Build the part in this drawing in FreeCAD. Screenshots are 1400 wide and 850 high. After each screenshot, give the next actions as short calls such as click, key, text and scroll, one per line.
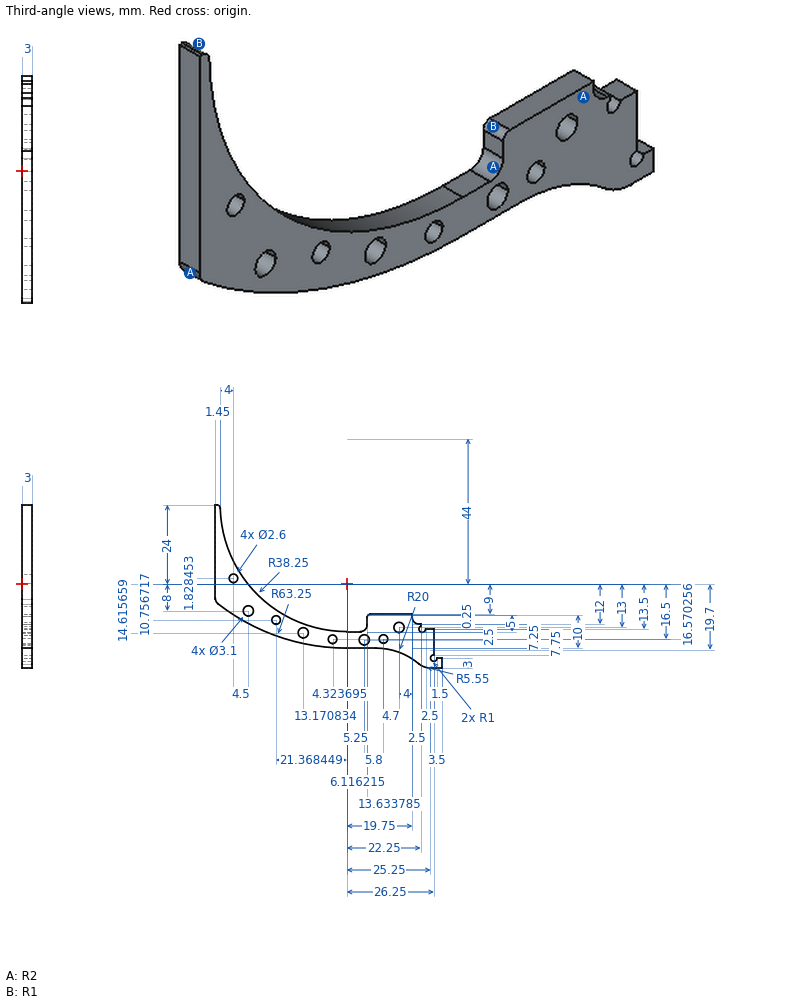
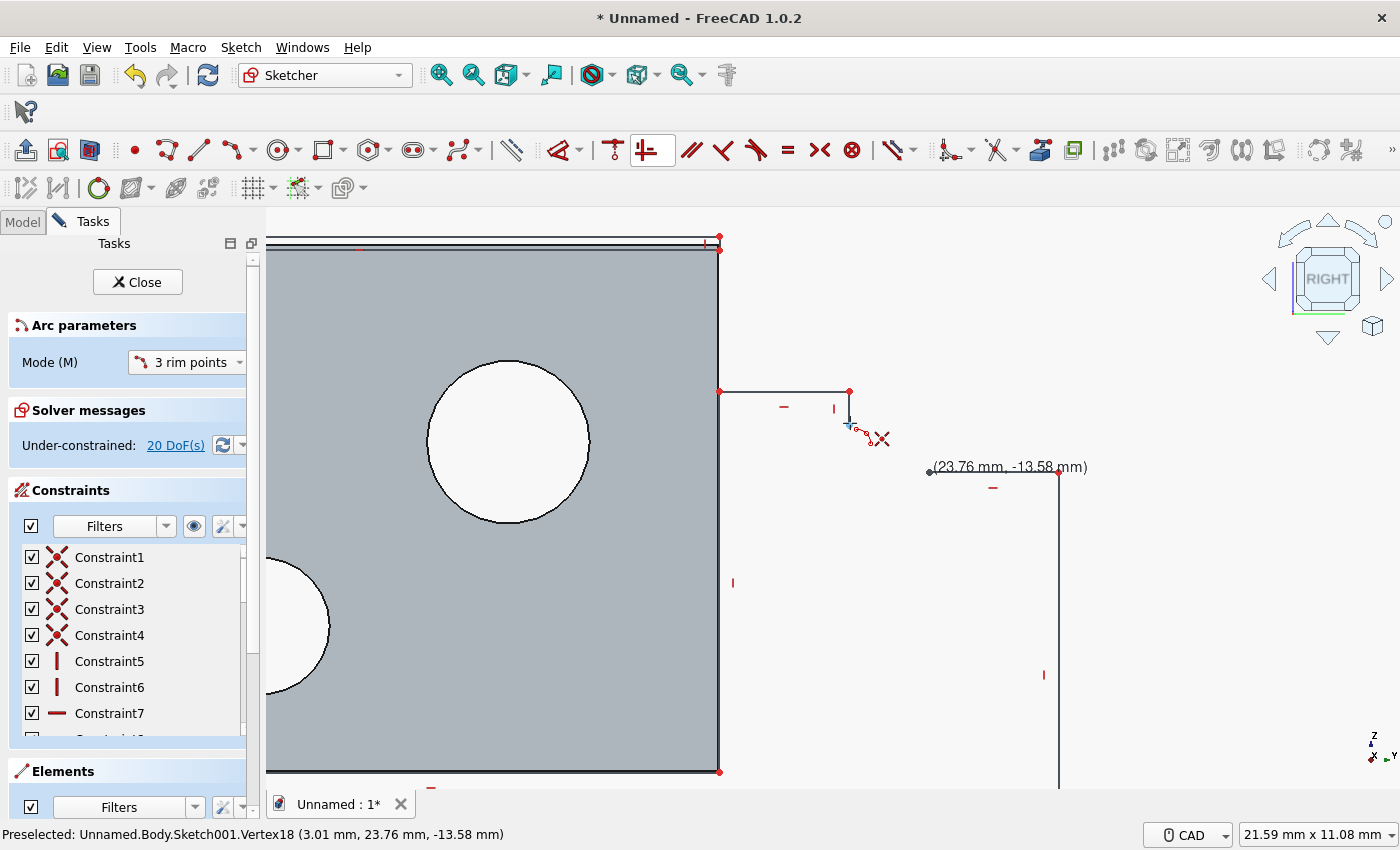
click(849, 426)
click(850, 514)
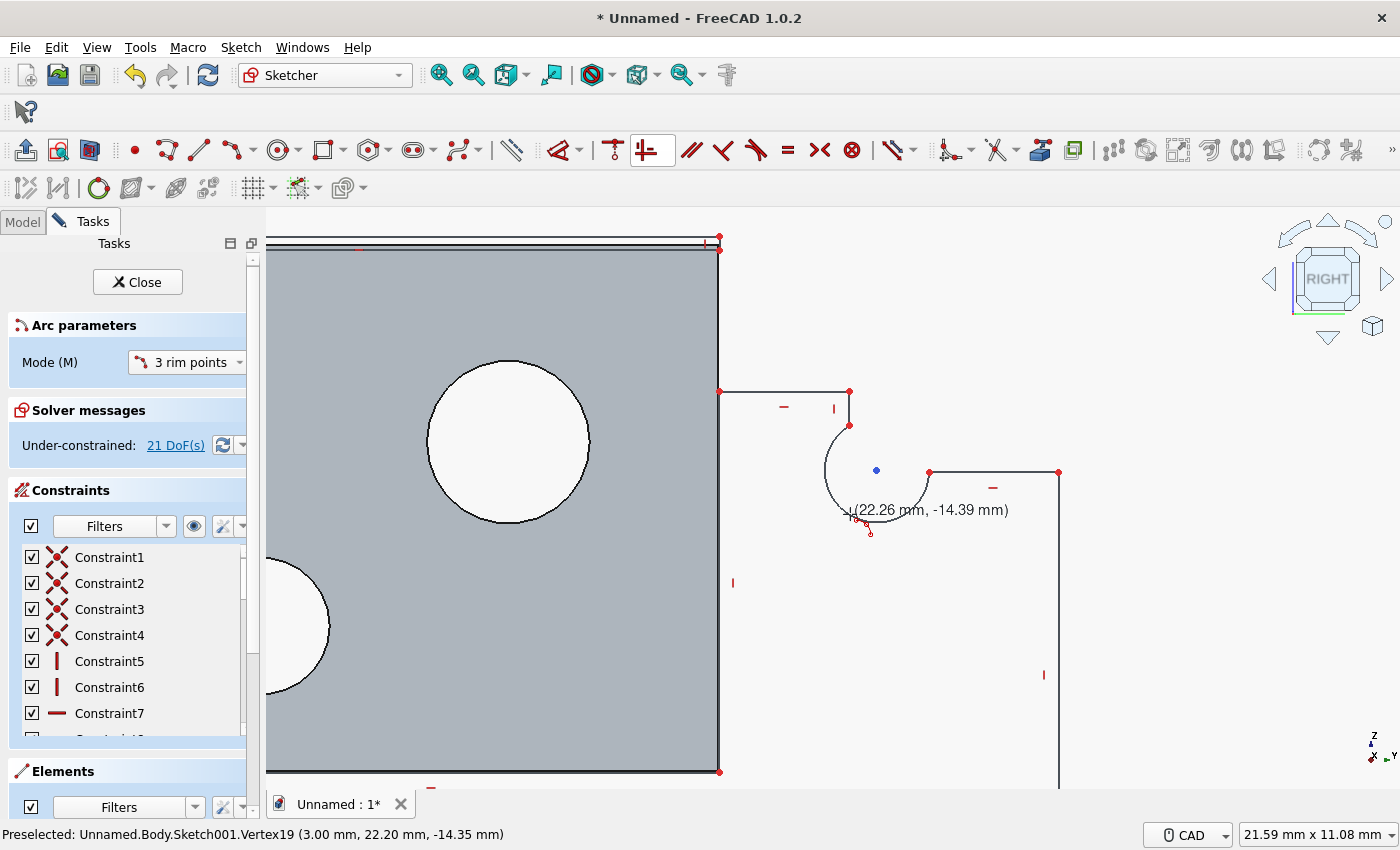
scroll(906, 531, down, 6)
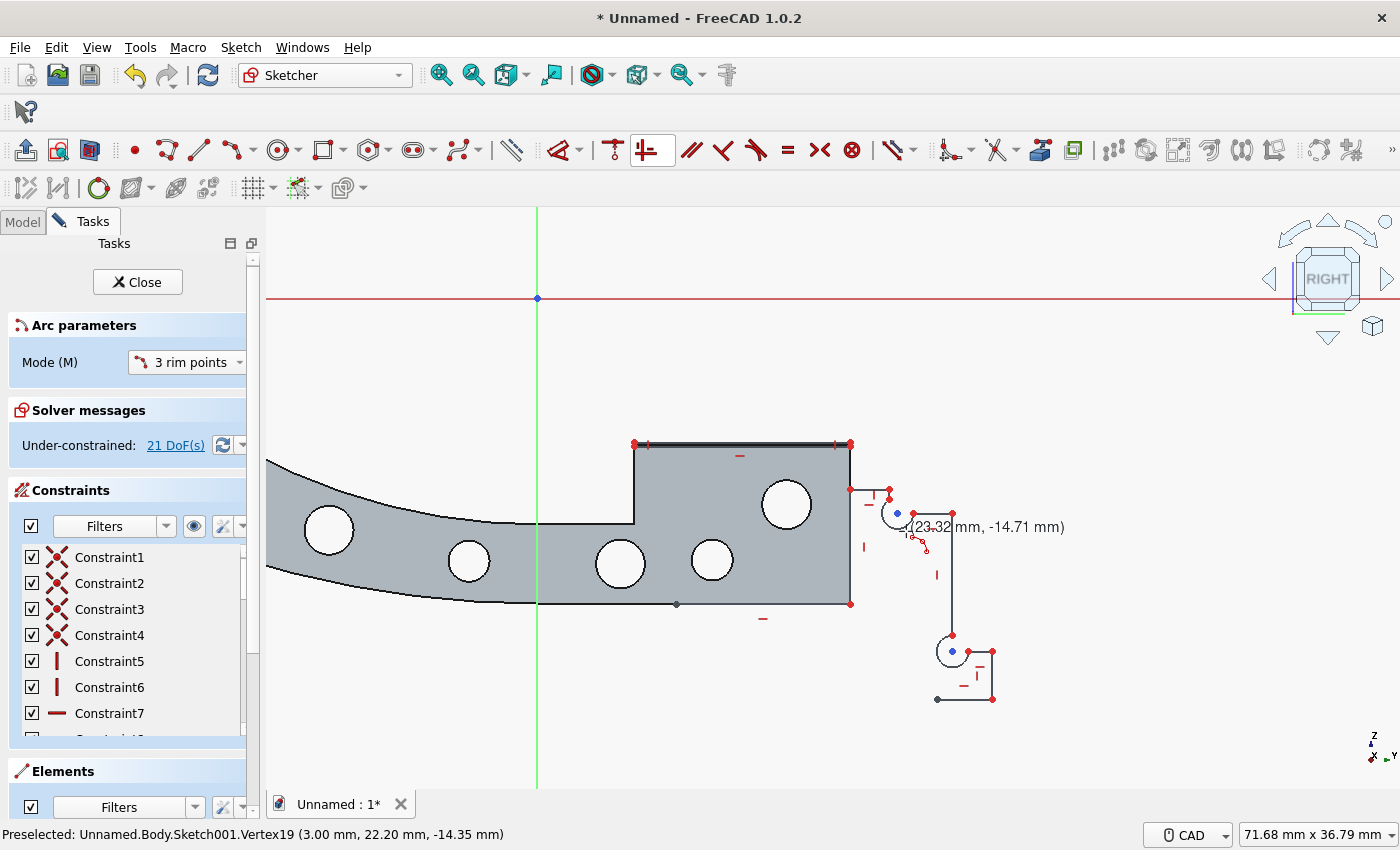
click(677, 604)
click(880, 678)
click(785, 623)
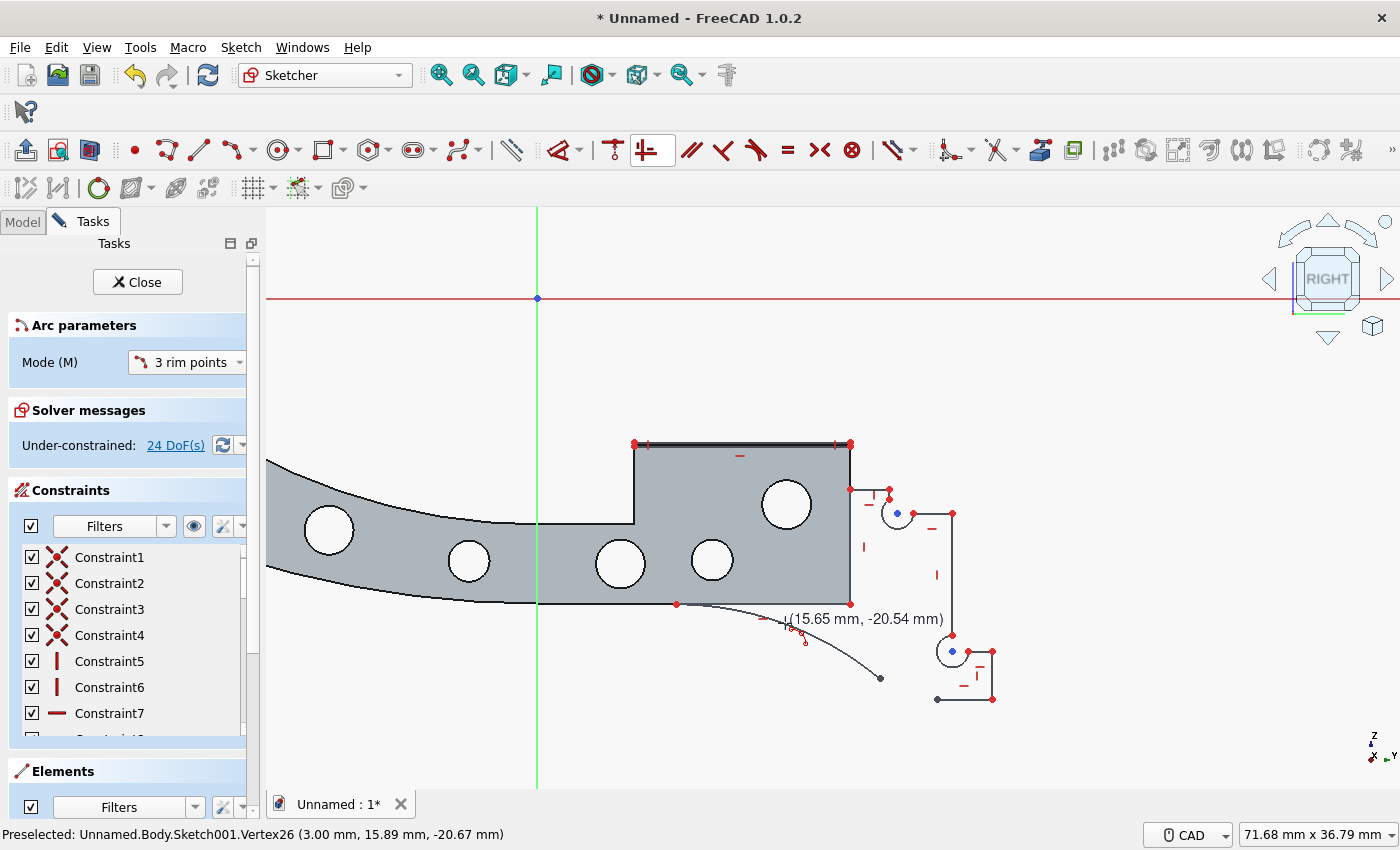
click(880, 679)
click(937, 700)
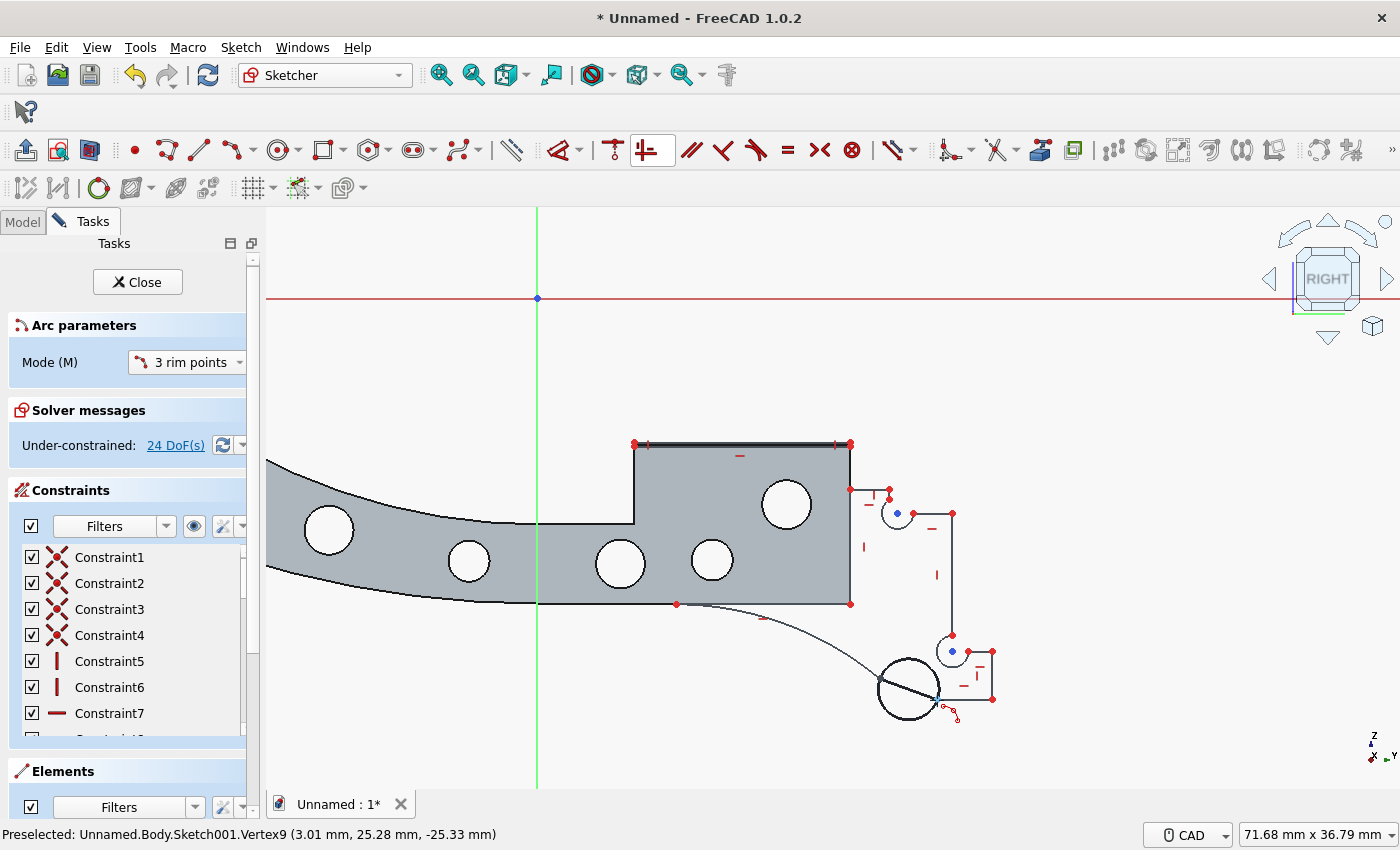
scroll(907, 693, up, 6)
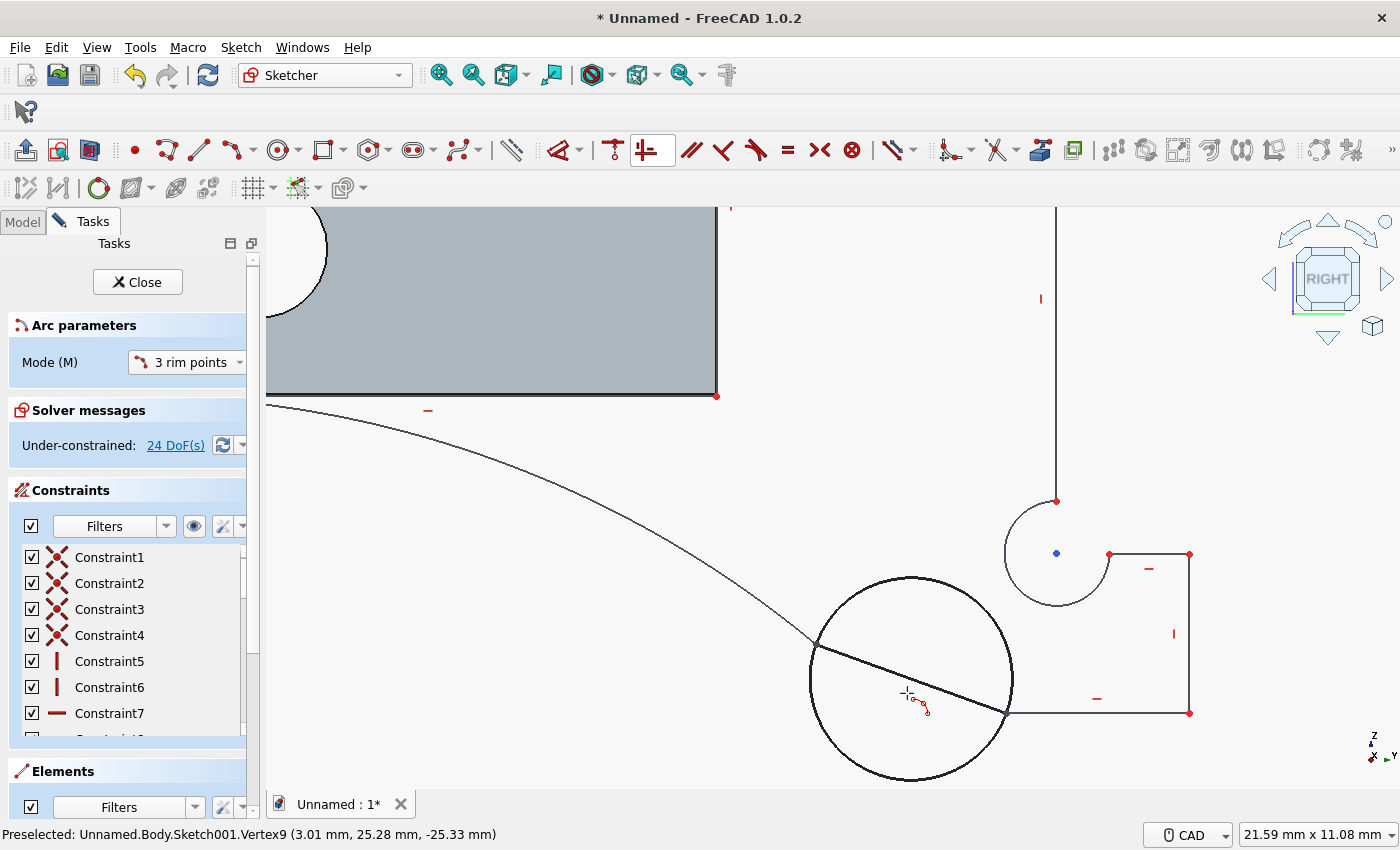
click(905, 692)
key(Escape)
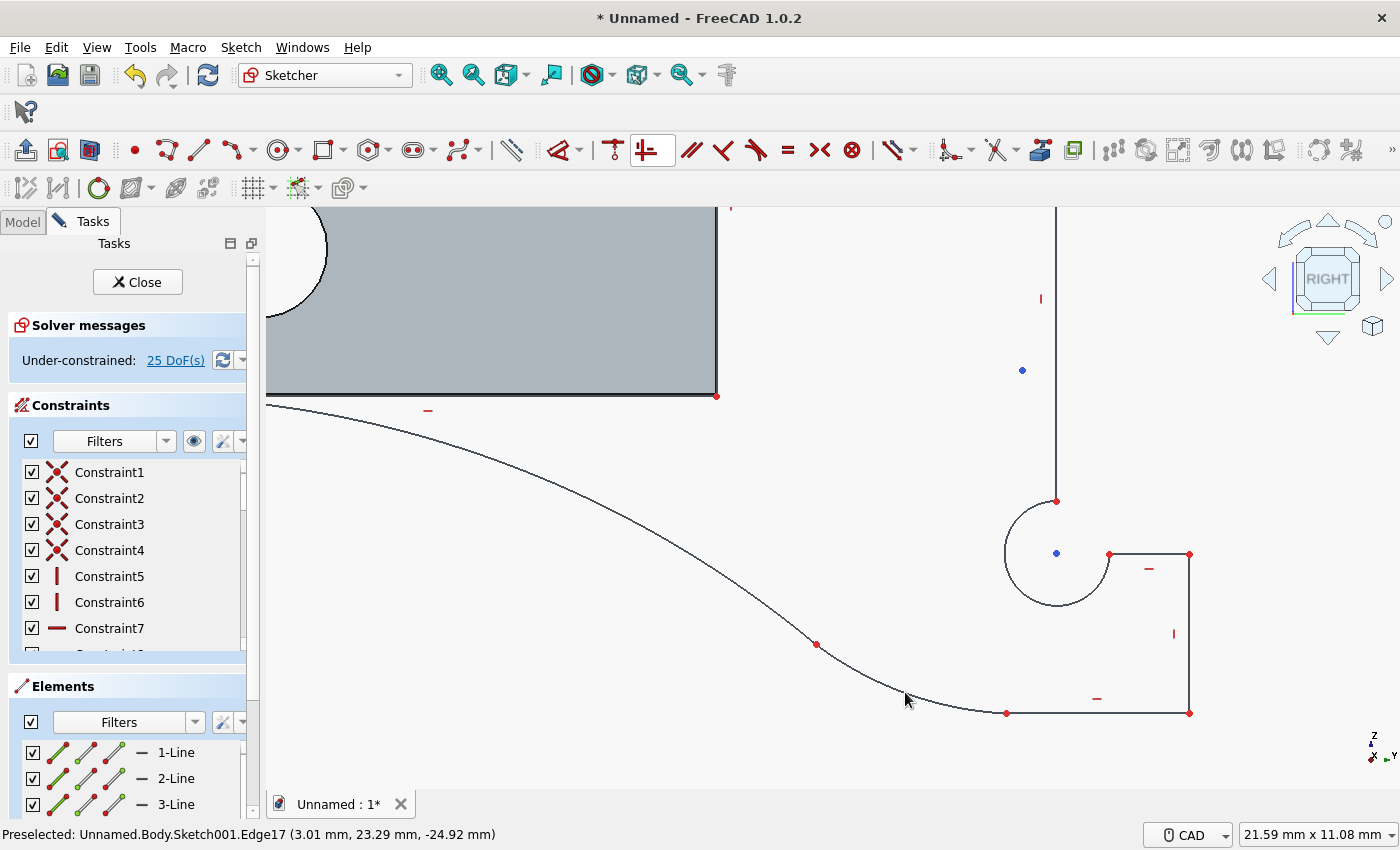
click(1061, 713)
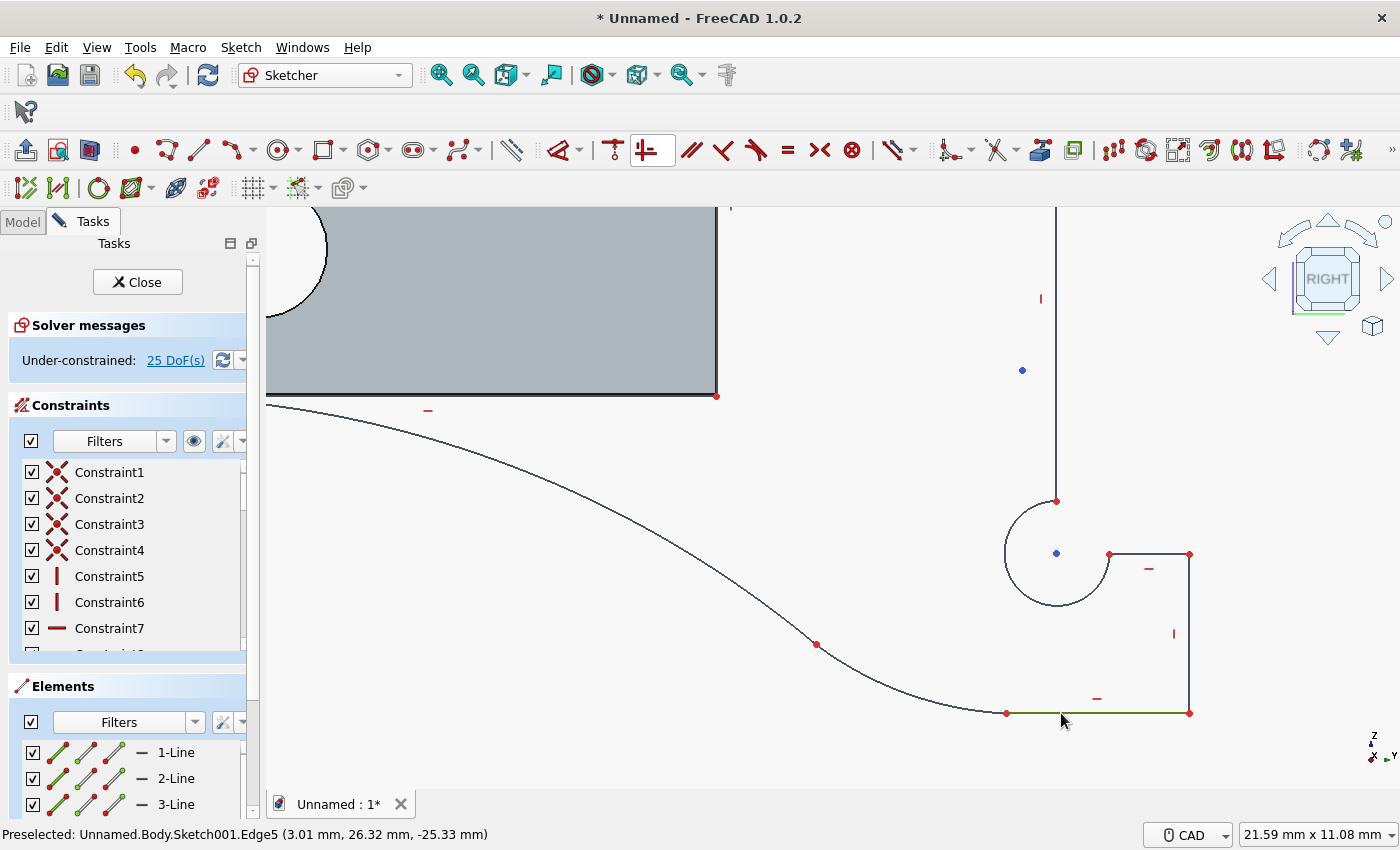
click(868, 677)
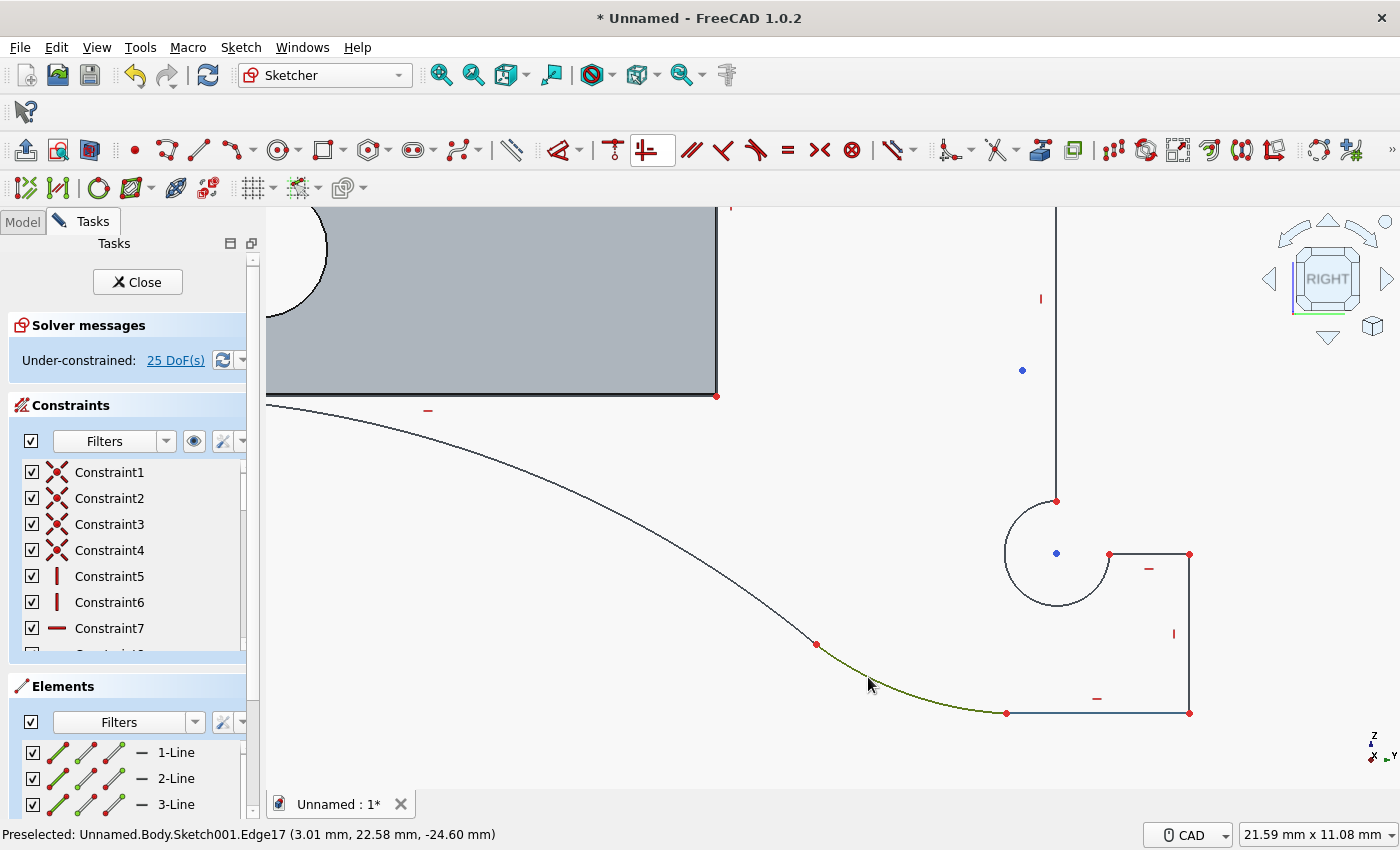
key(t)